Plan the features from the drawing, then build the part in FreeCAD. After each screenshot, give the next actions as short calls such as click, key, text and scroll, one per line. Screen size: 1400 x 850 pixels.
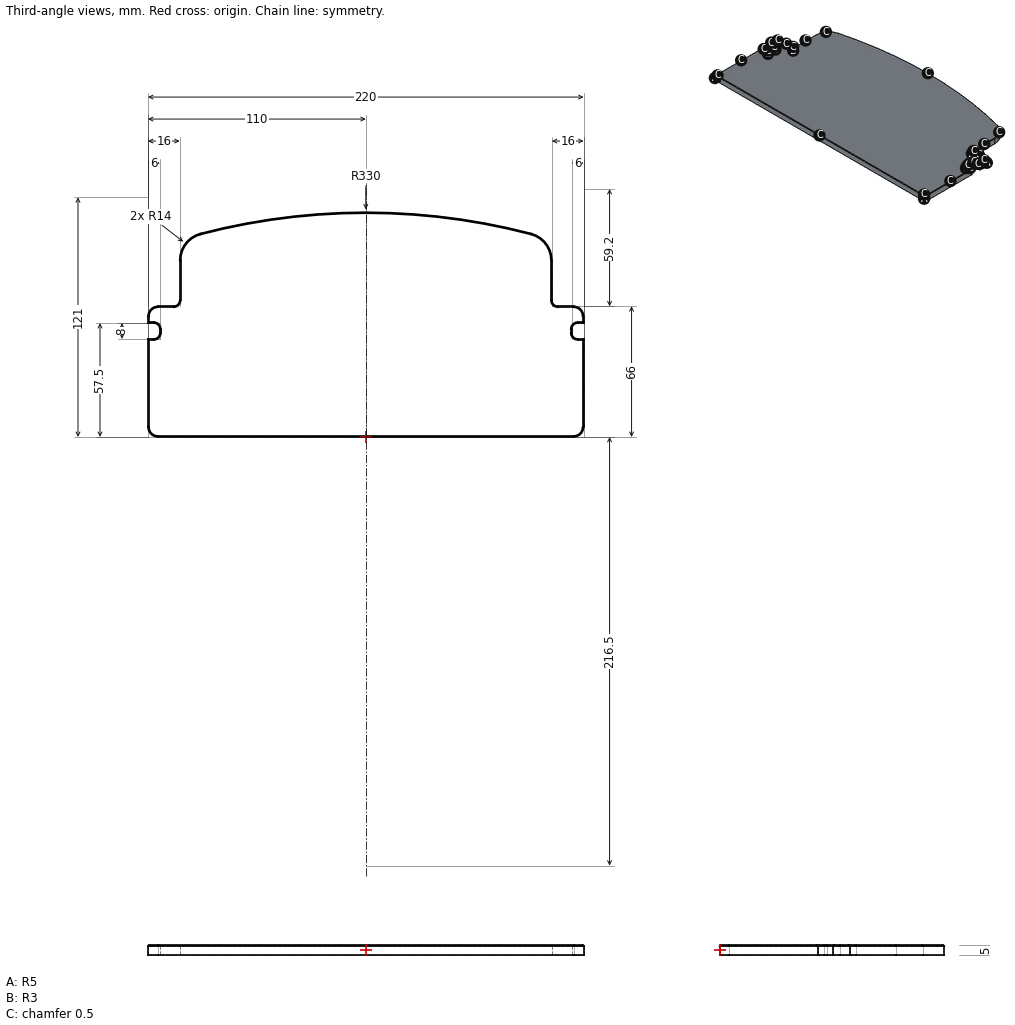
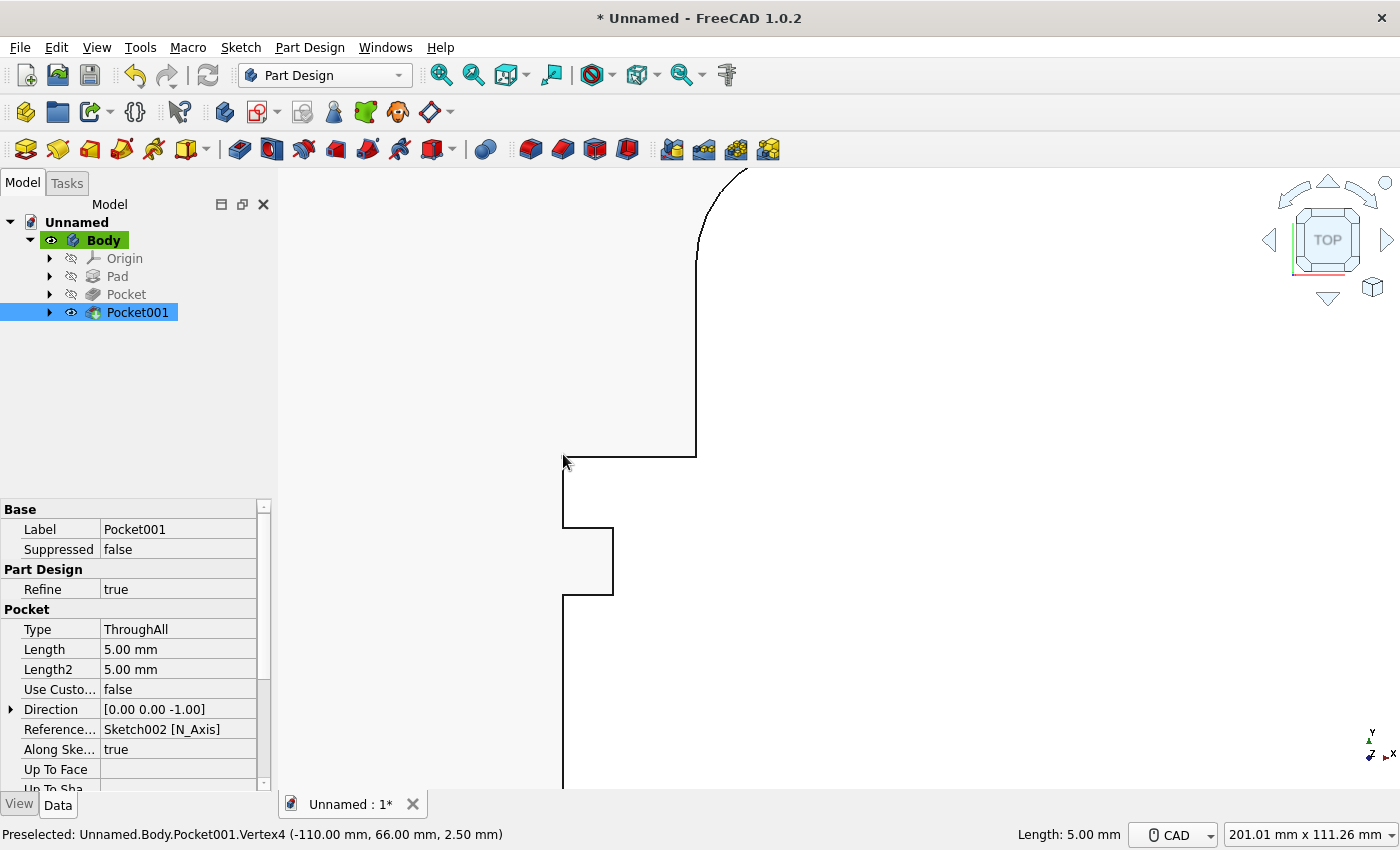
key(v)
key(f)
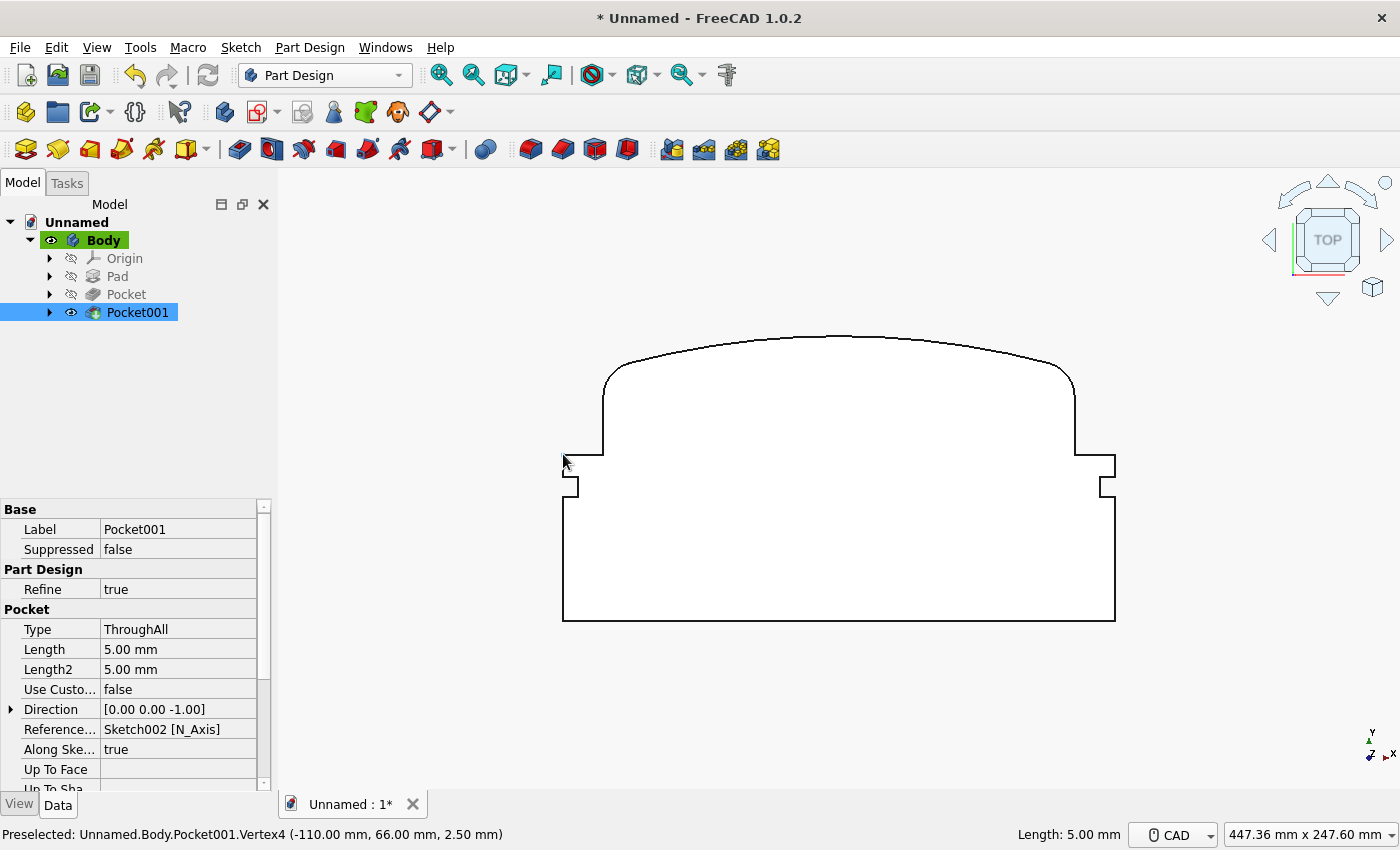
key(1)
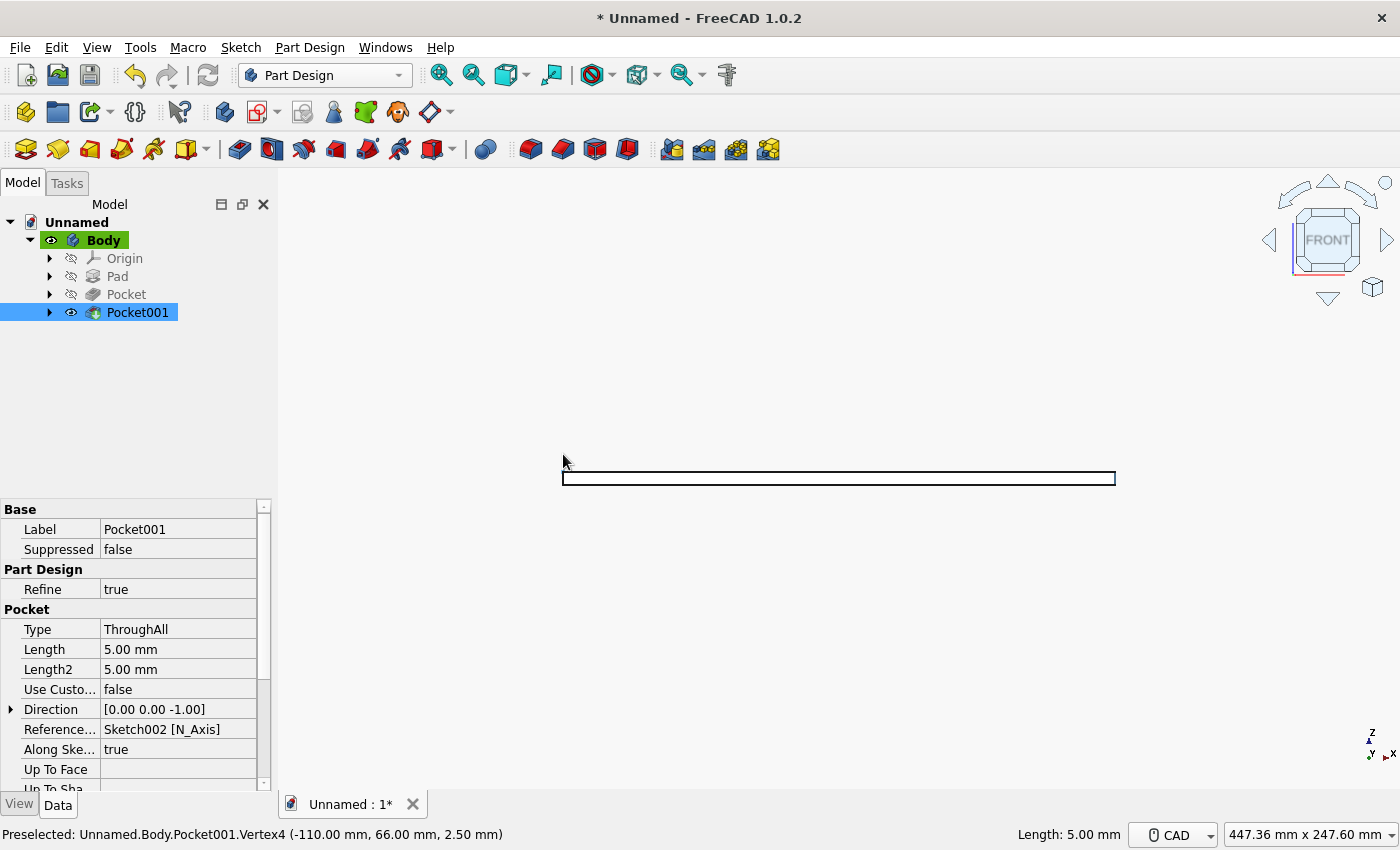
scroll(563, 477, up, 6)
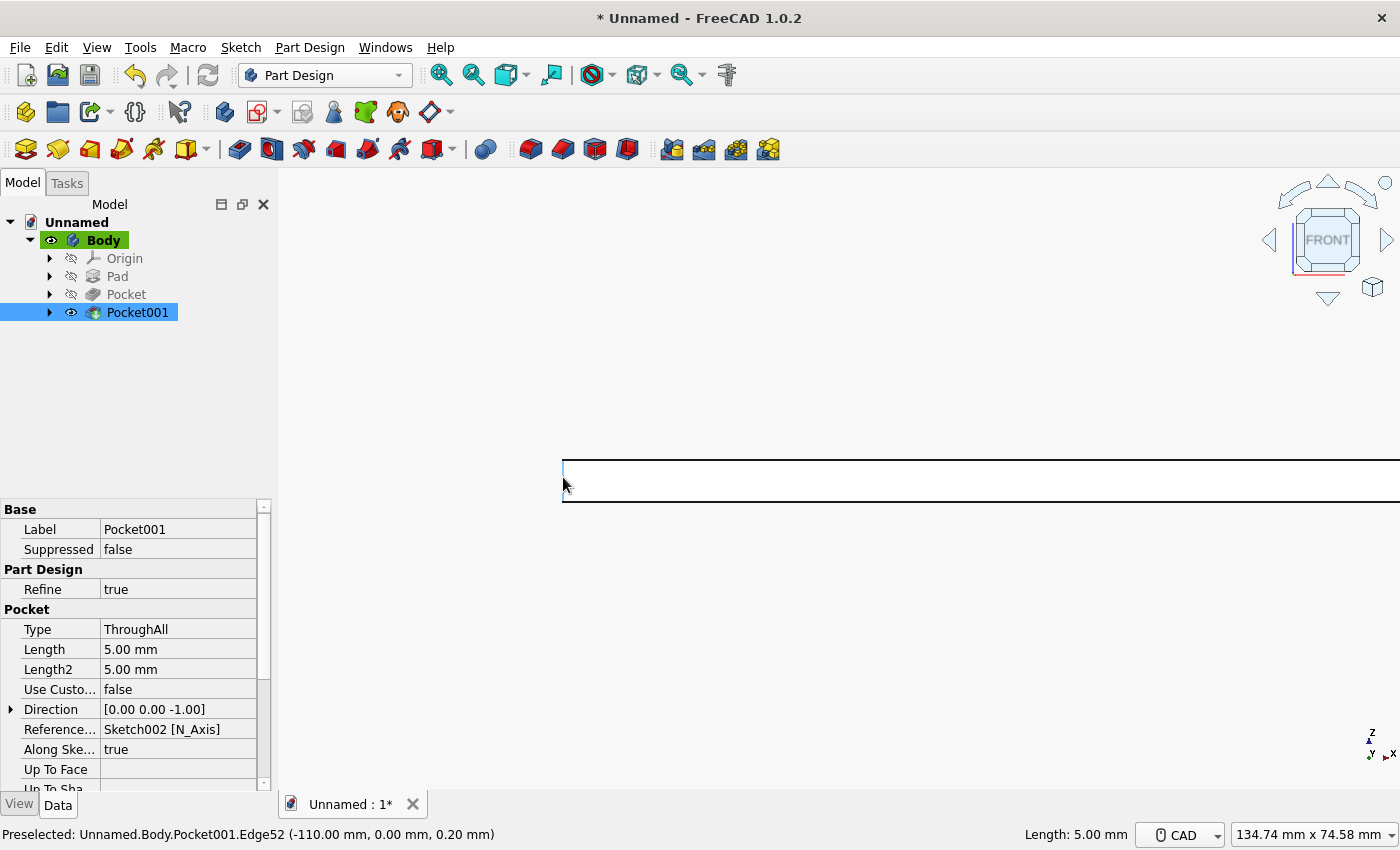
click(563, 480, ctrl)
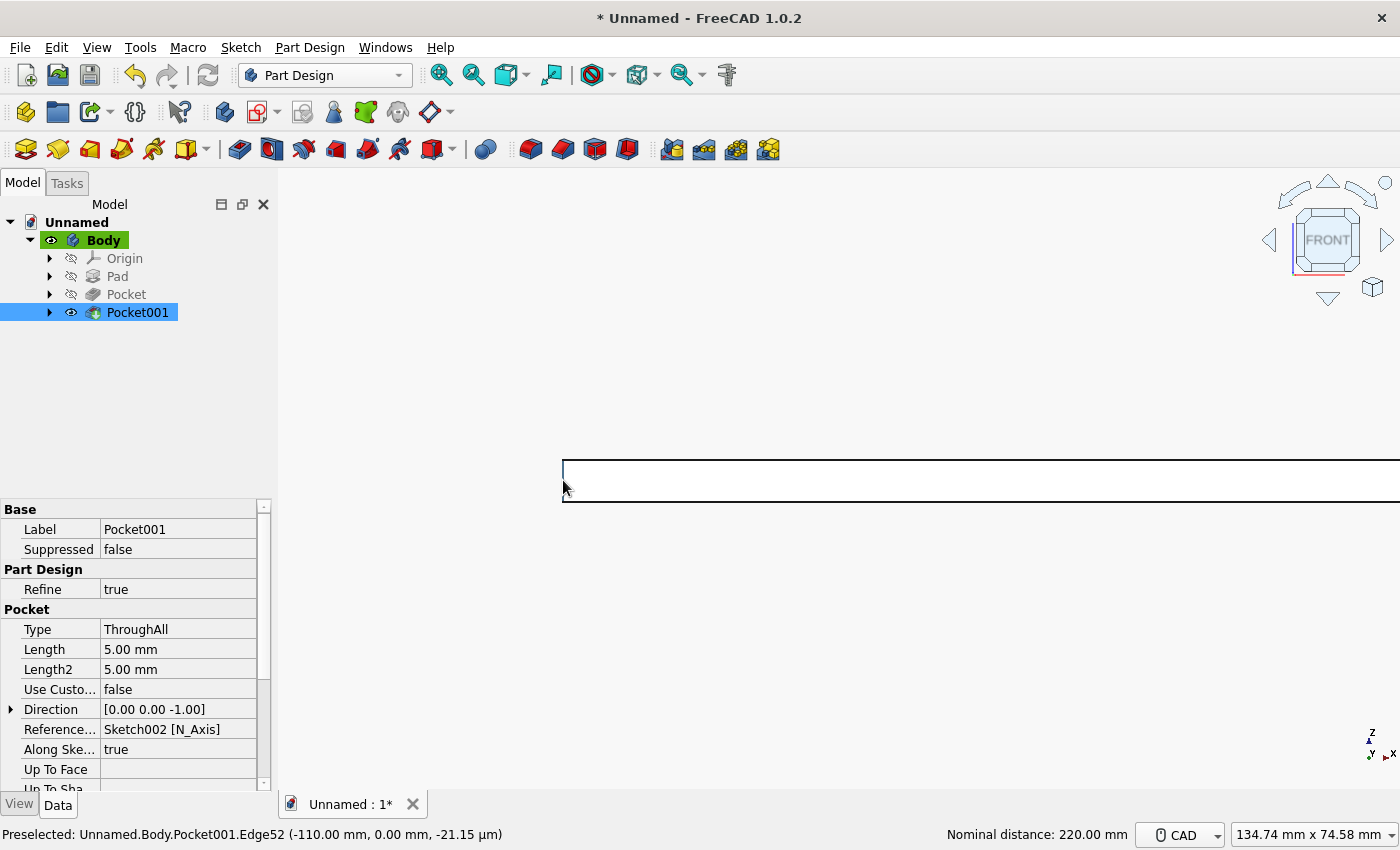
key(v)
key(f)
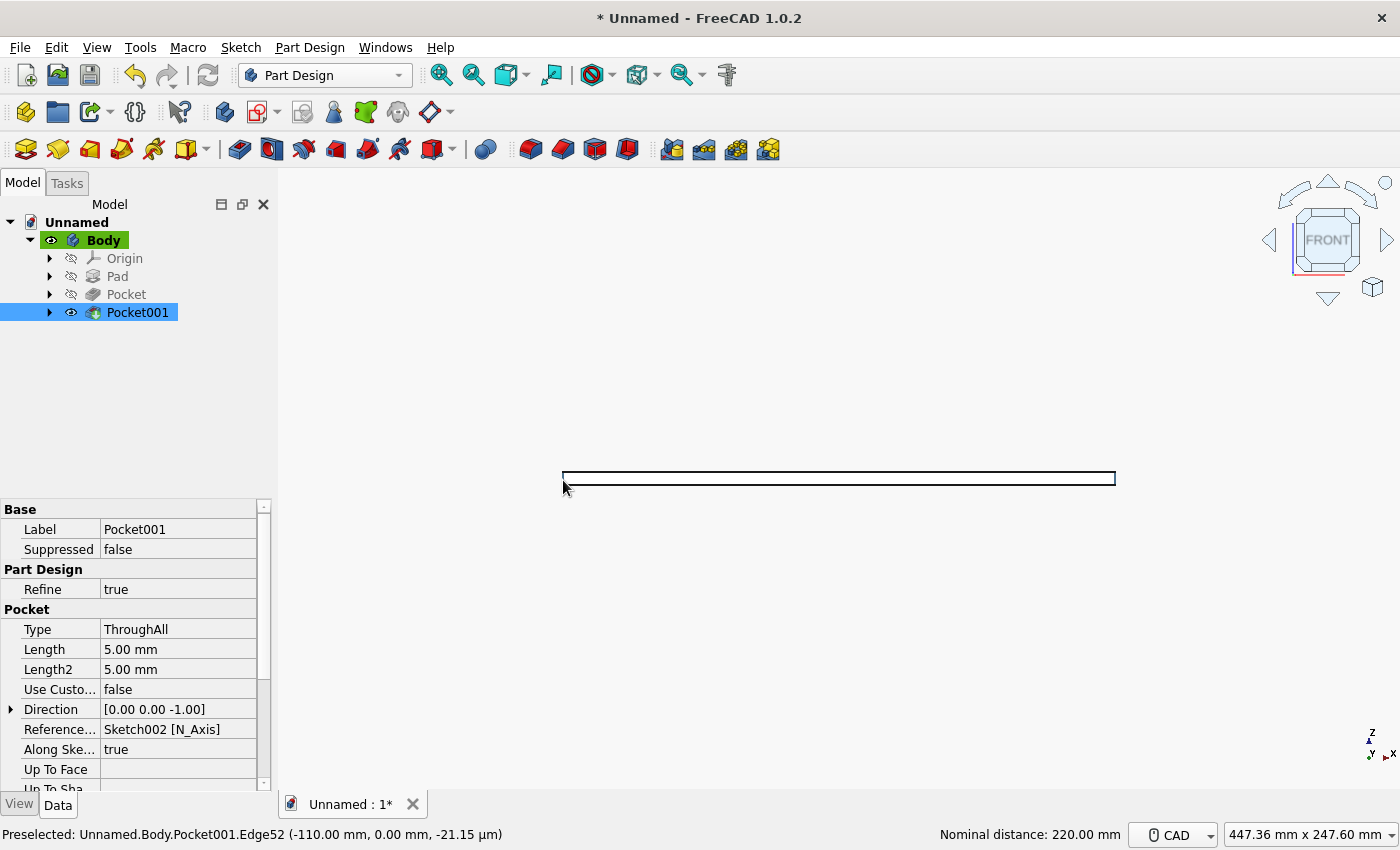
key(3)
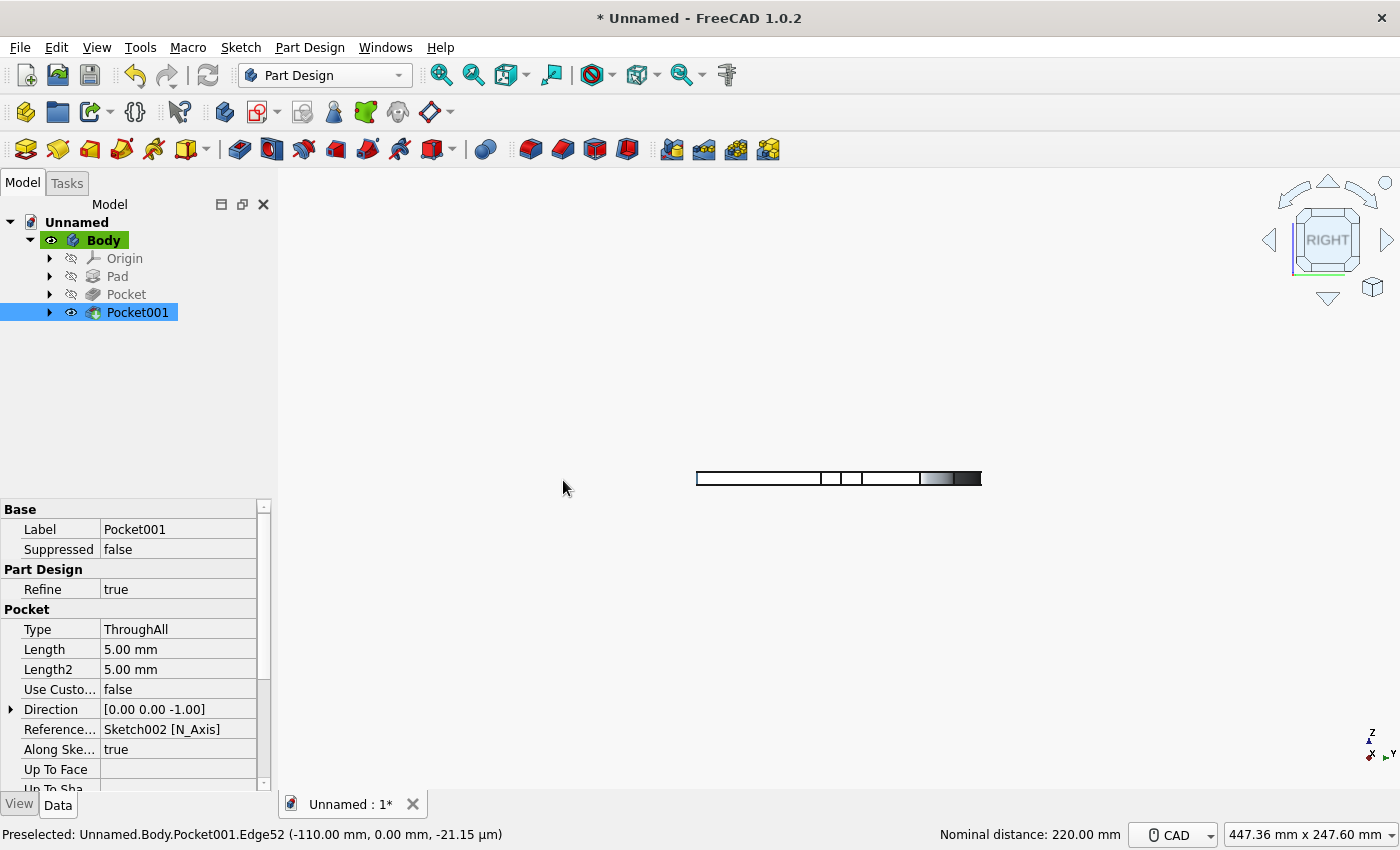
key(v)
key(f)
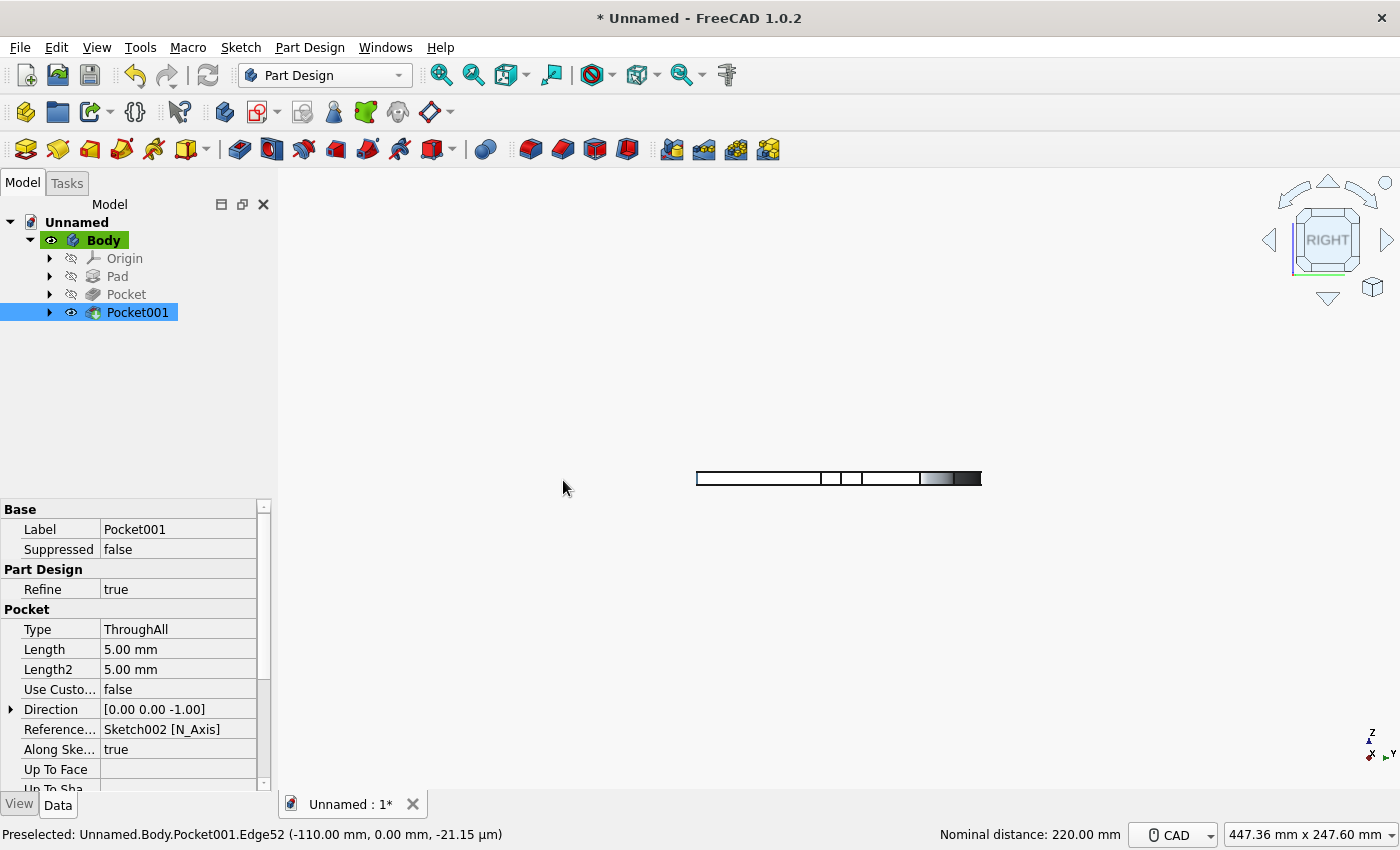
scroll(862, 477, up, 6)